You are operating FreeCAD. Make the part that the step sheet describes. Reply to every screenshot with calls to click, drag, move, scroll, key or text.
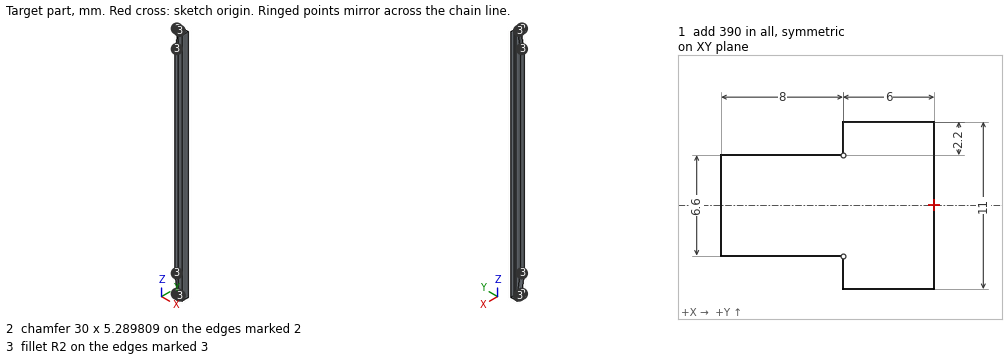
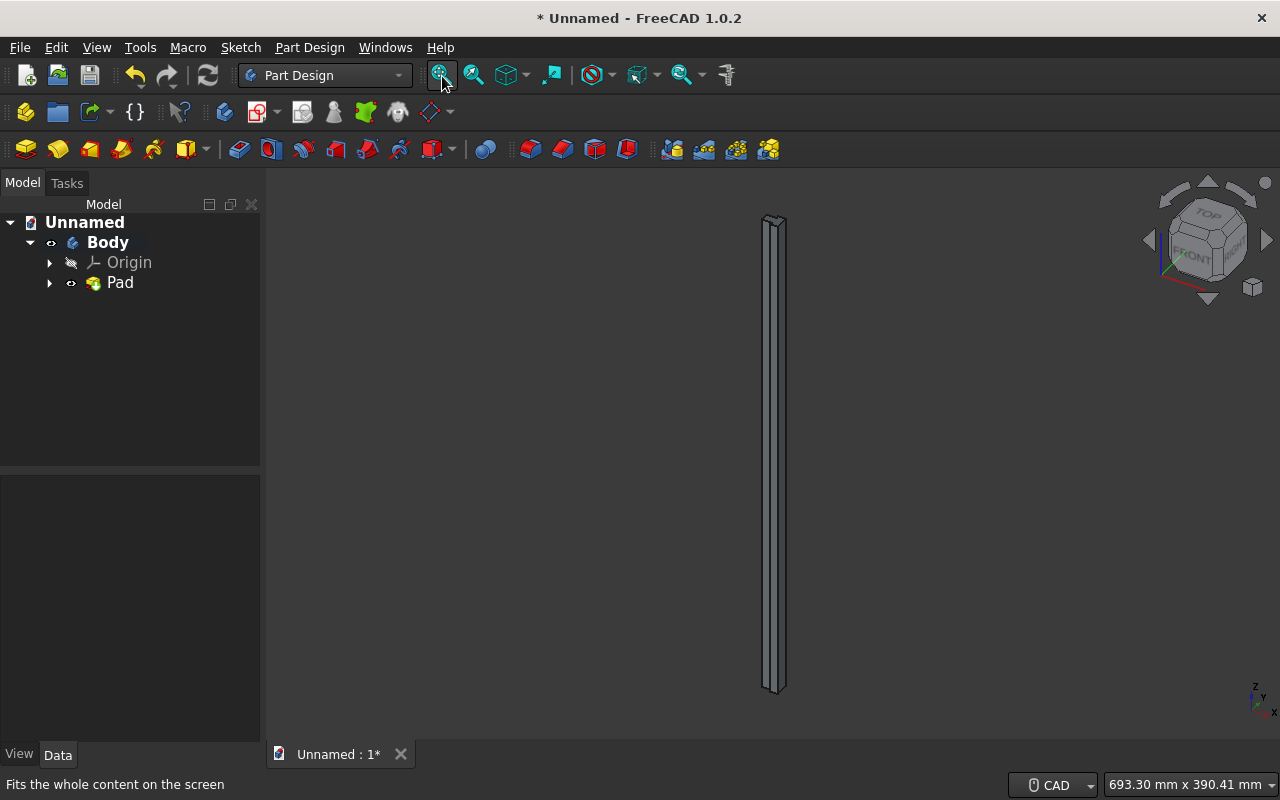
key(0)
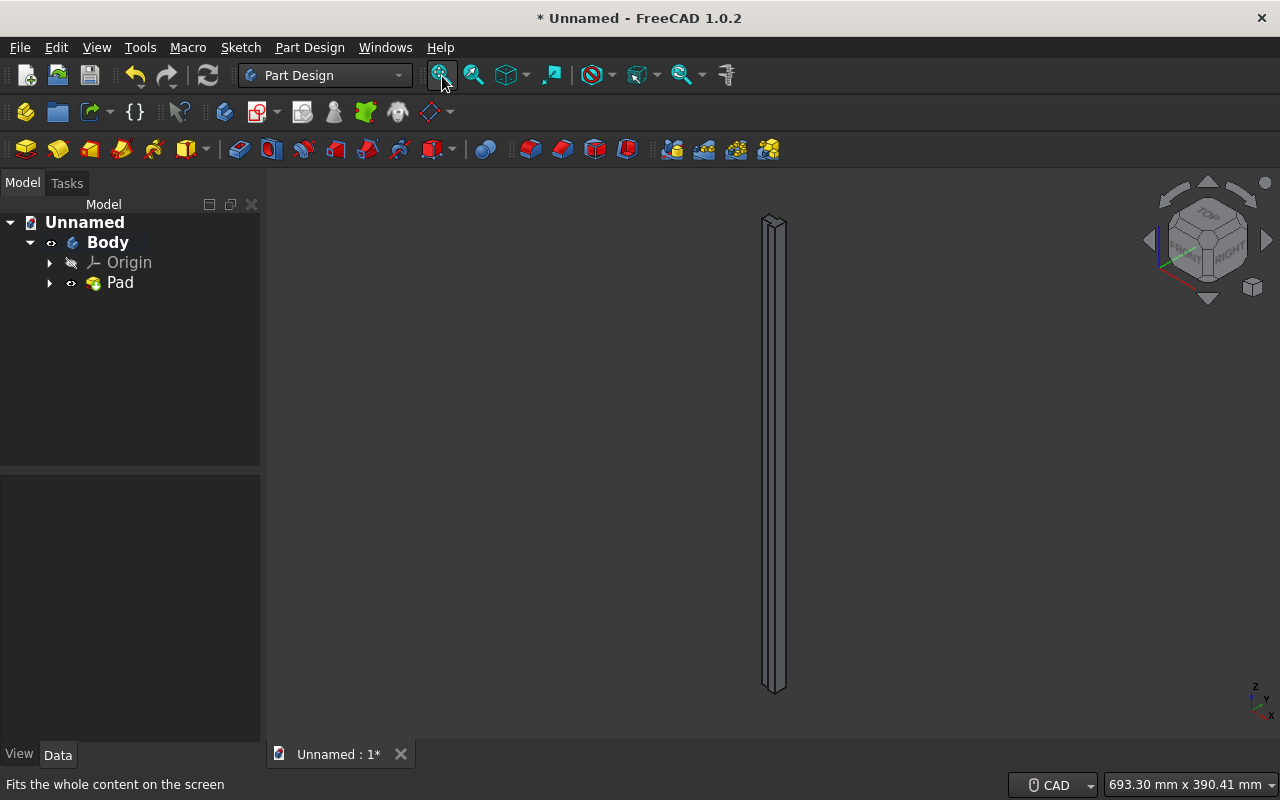
scroll(766, 215, up, 8)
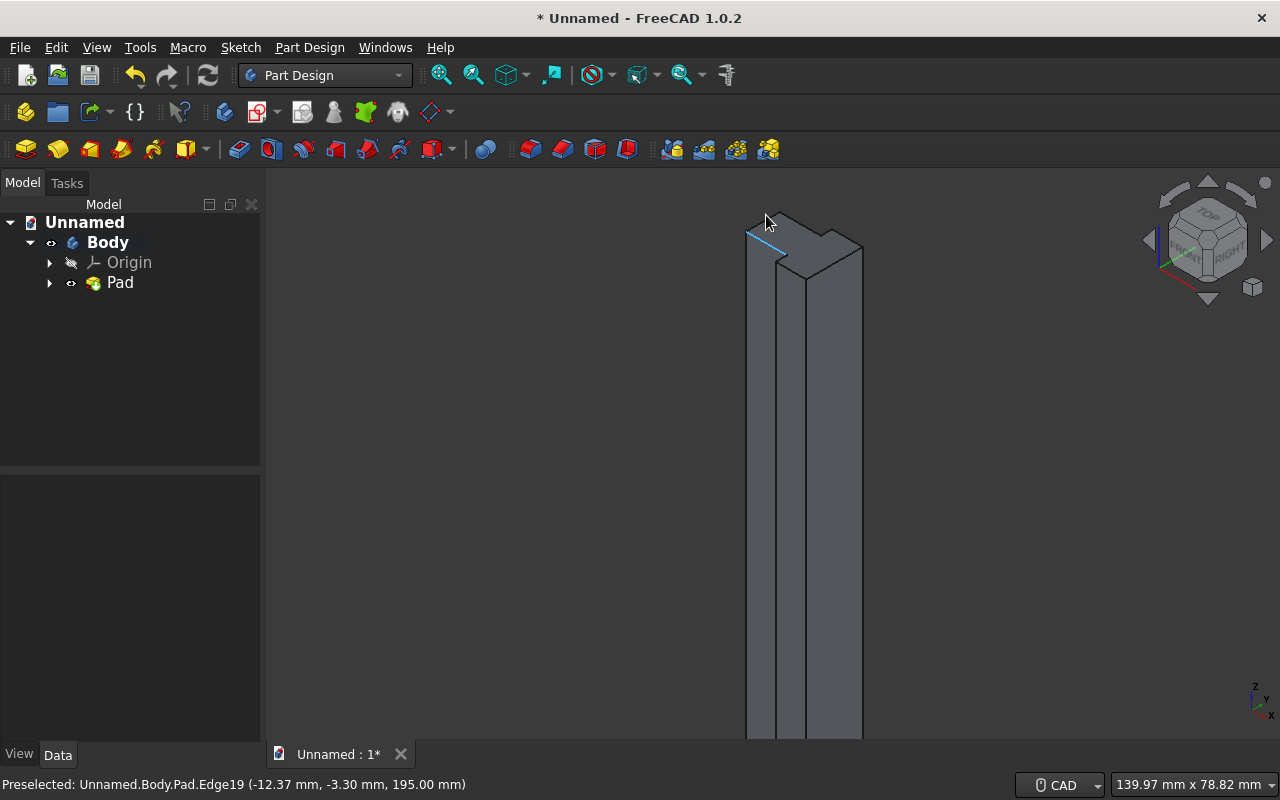
click(442, 76)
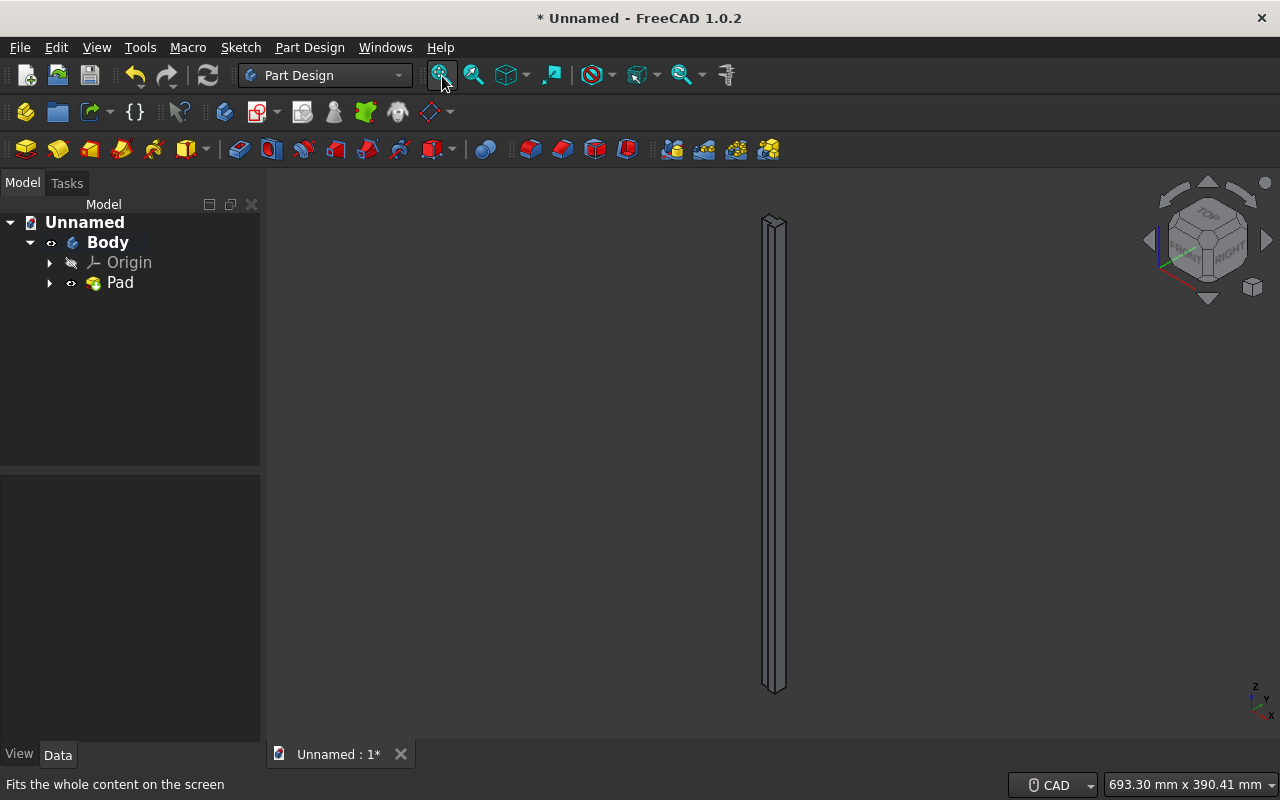
key(2)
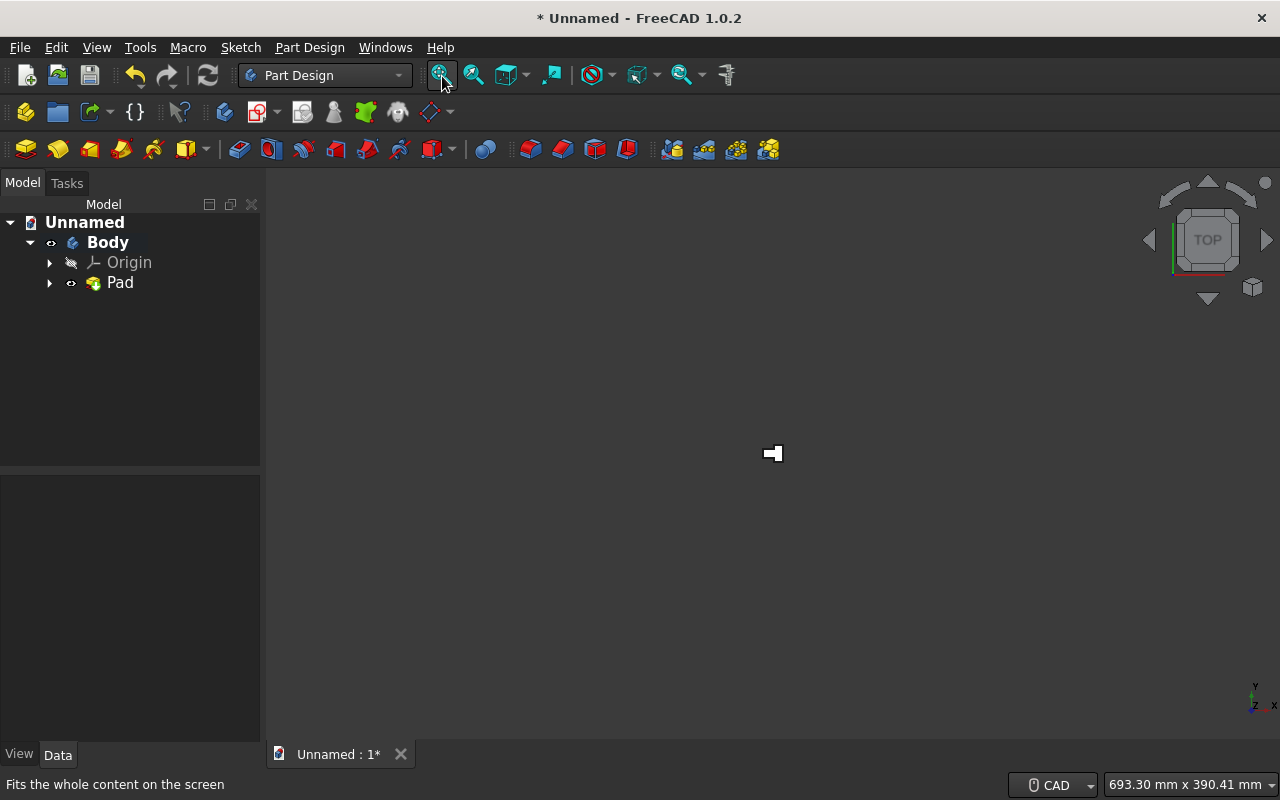
click(442, 76)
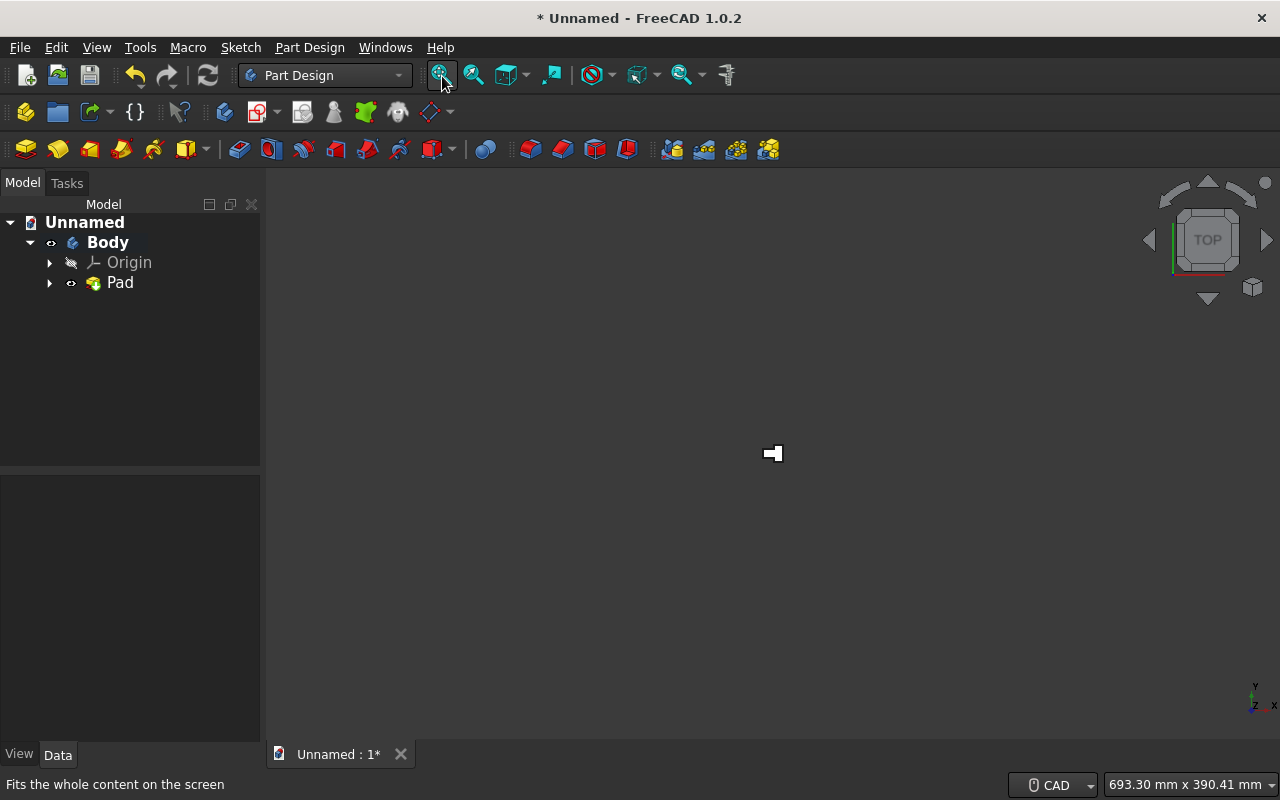
scroll(763, 452, up, 8)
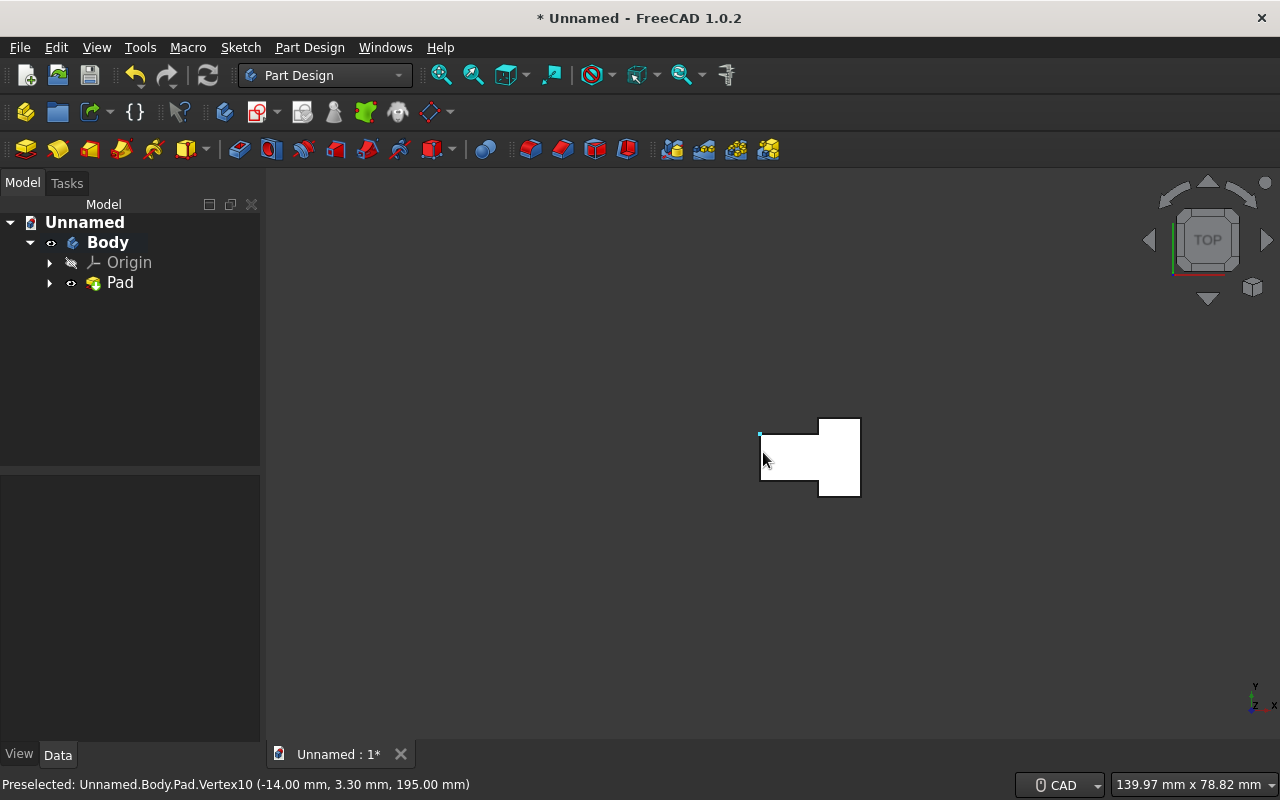
click(760, 456)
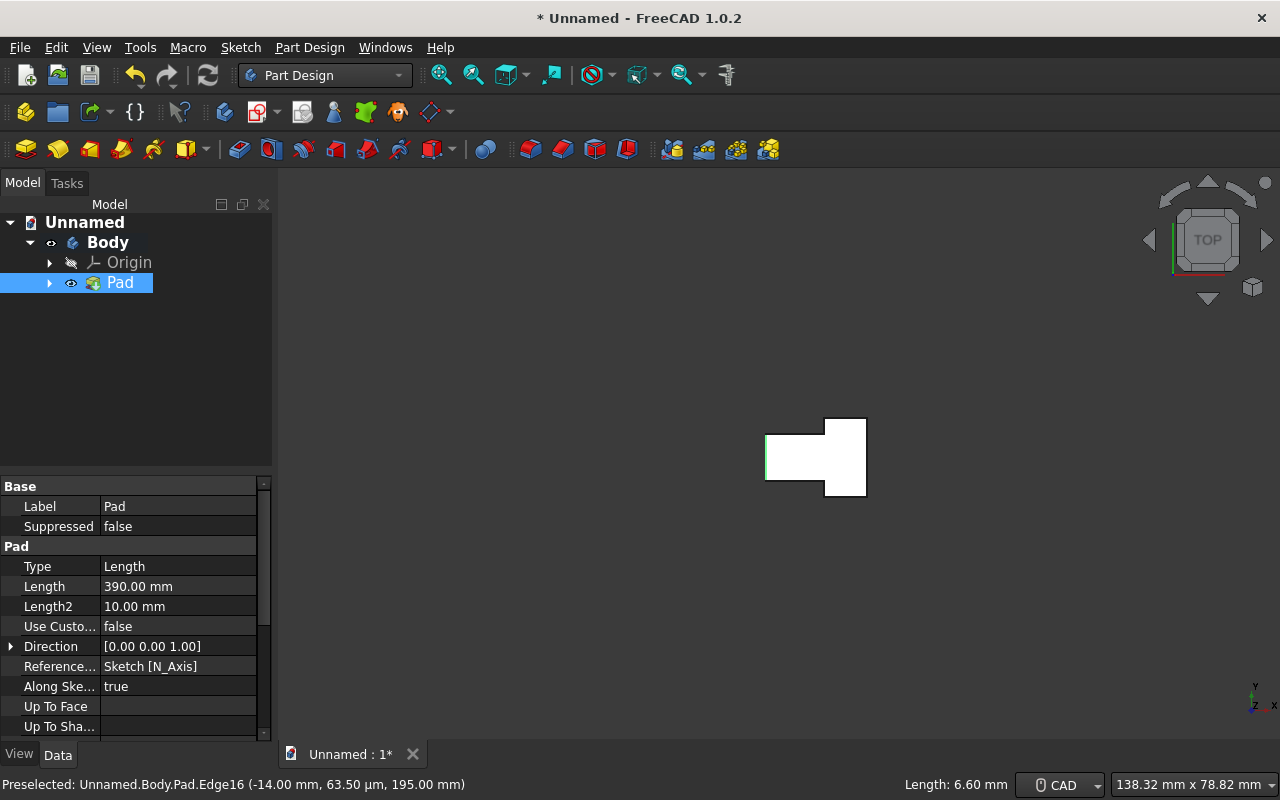
click(442, 76)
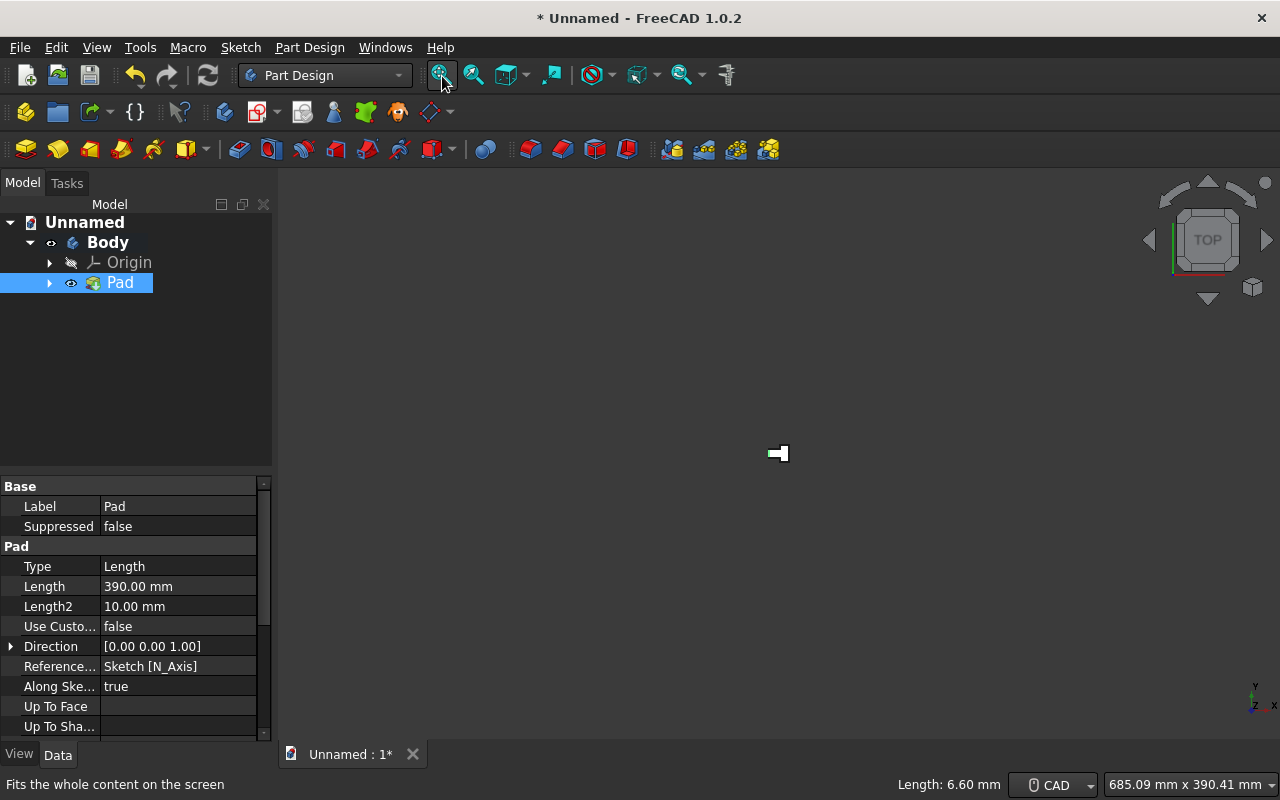
key(1)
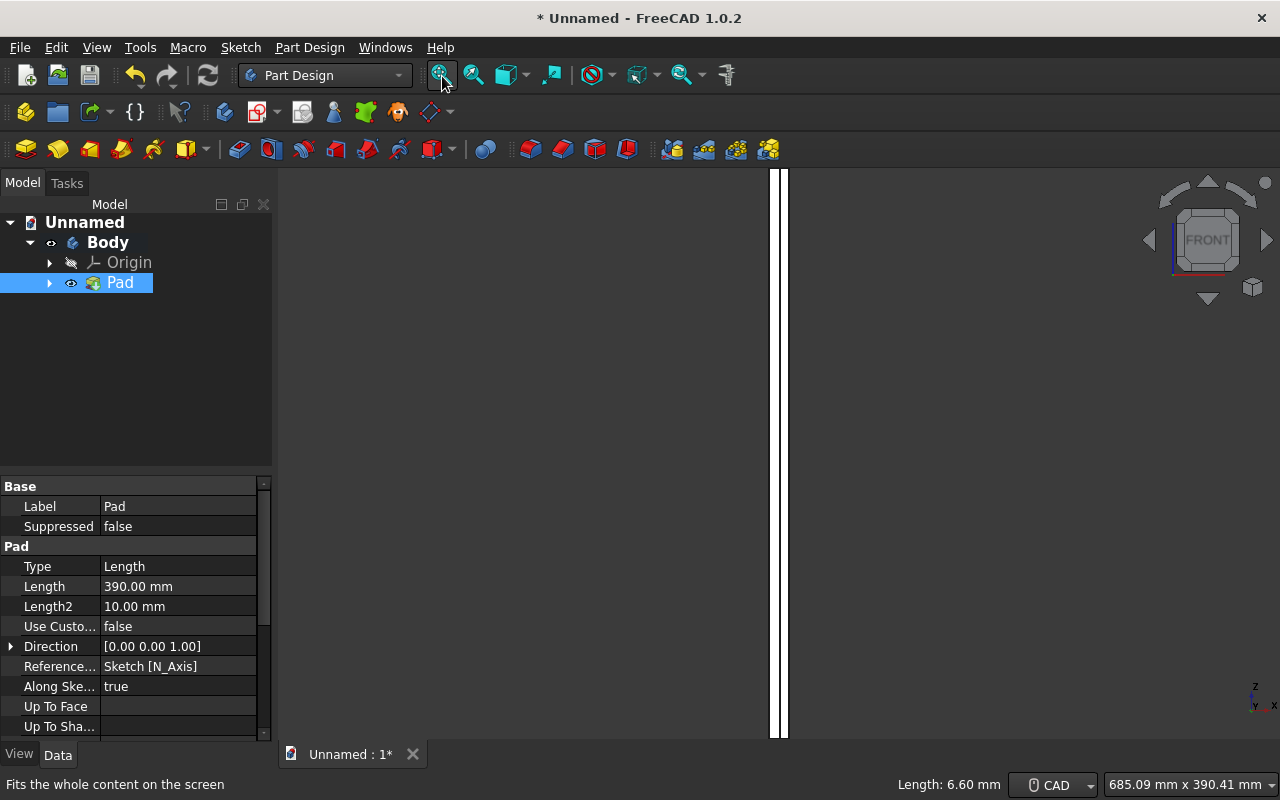
click(442, 76)